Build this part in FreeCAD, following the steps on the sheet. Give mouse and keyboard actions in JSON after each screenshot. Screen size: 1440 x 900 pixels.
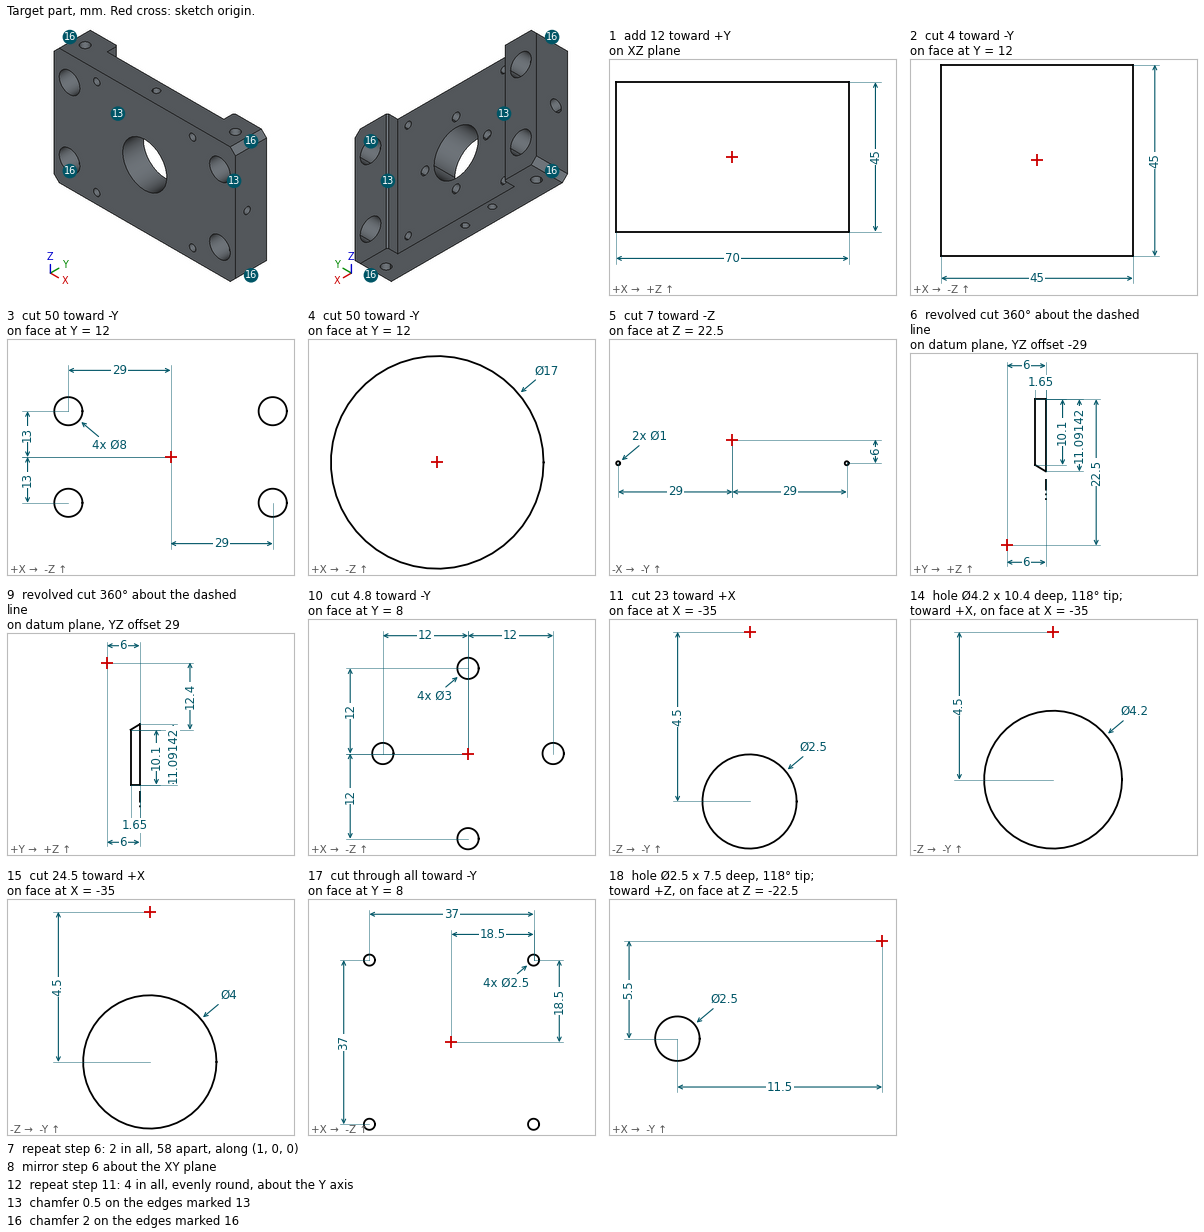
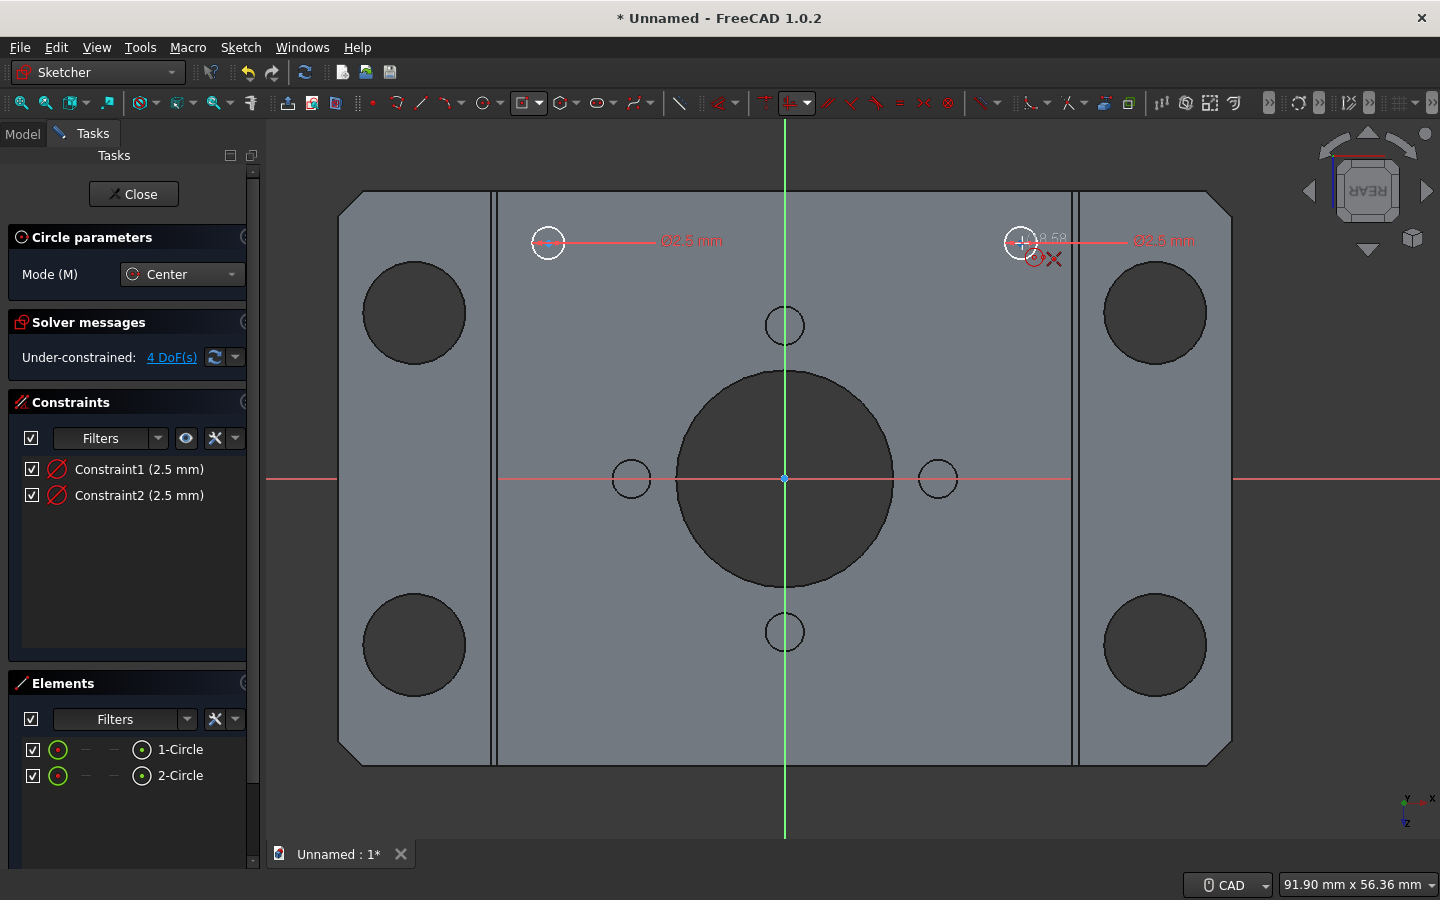
{"action": "scroll", "coordinate": [548, 715], "scroll_direction": "up", "scroll_amount": 2}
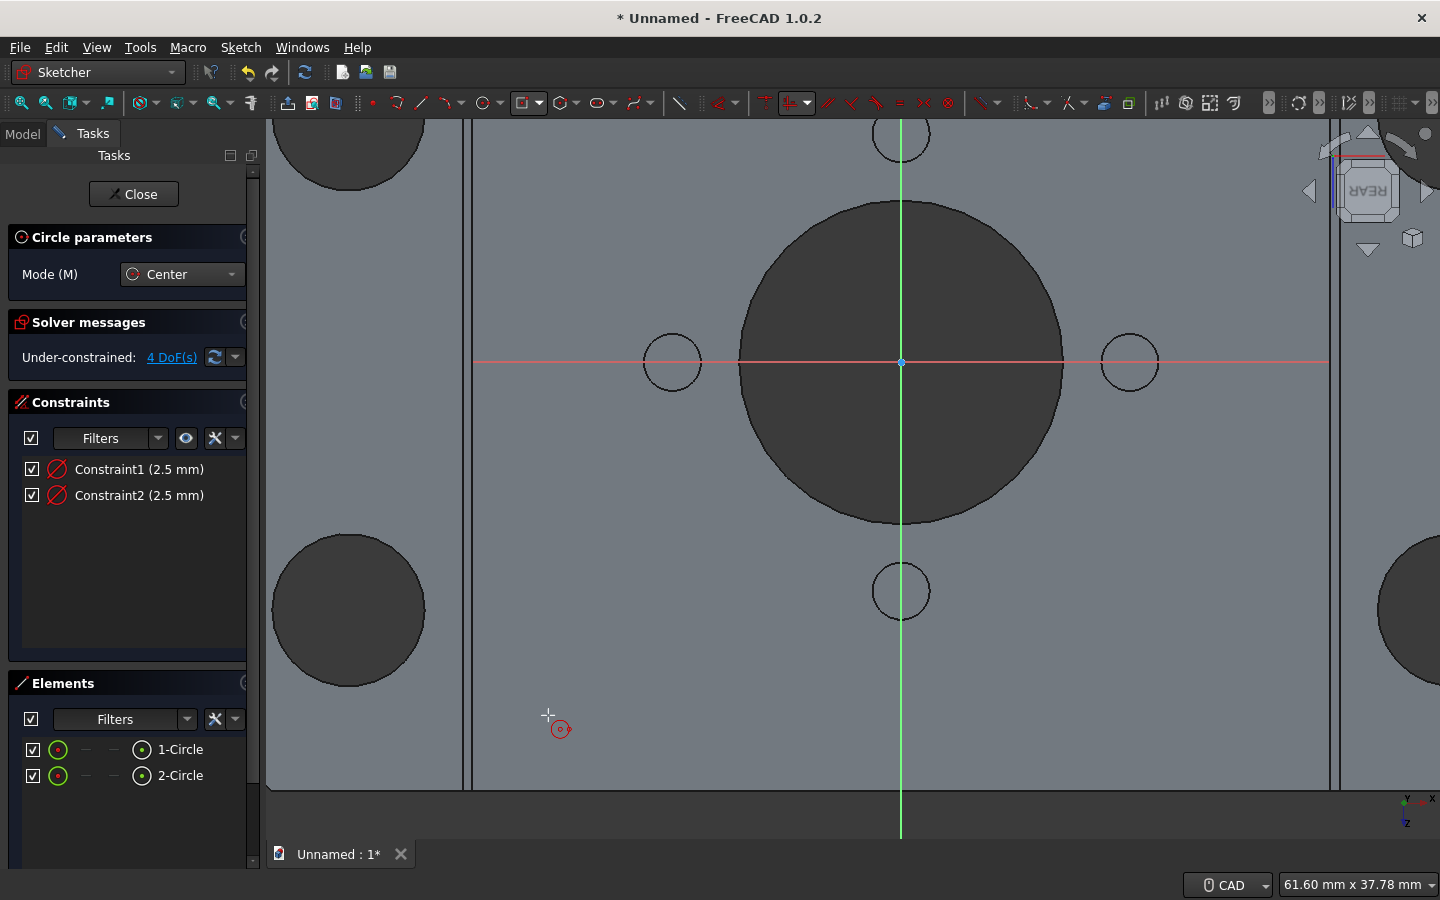
{"action": "left_click", "coordinate": [549, 715]}
{"action": "mouse_move", "coordinate": [565, 698]}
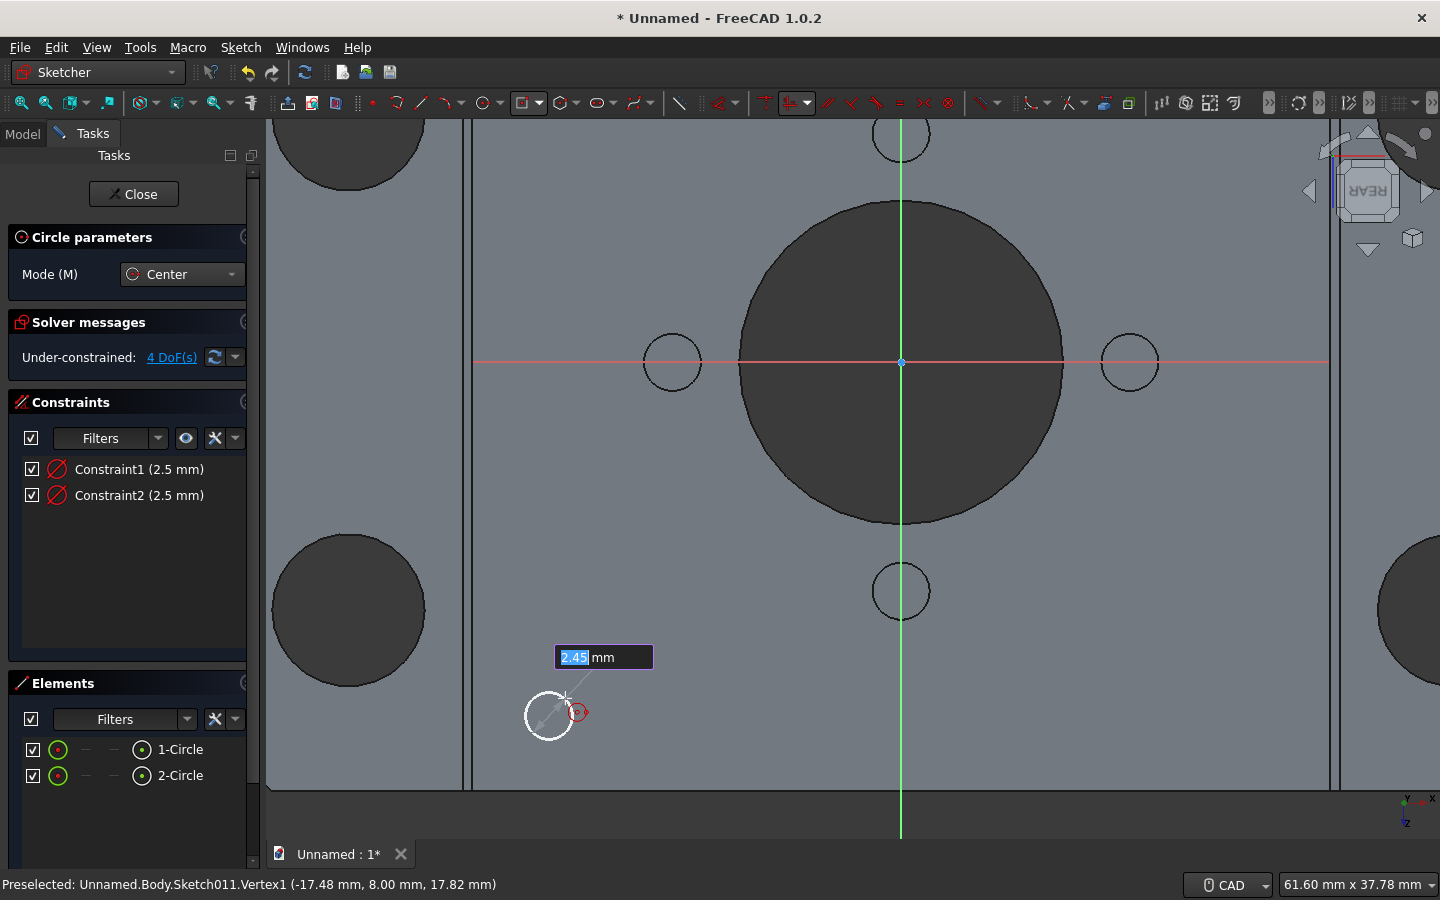
{"action": "type", "text": "2.5"}
{"action": "key", "text": "Return"}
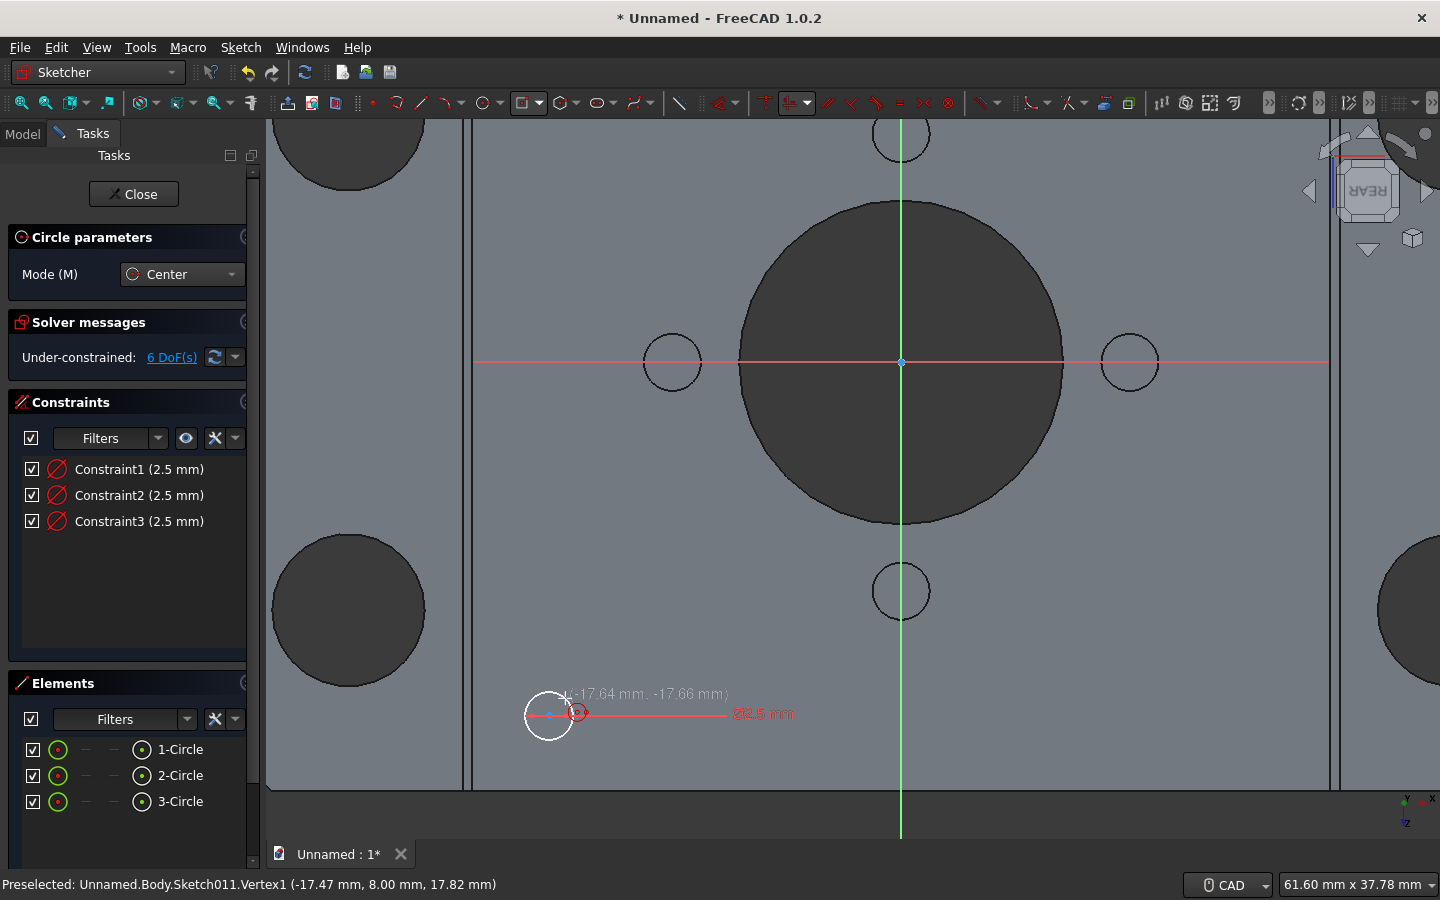
{"action": "left_click", "coordinate": [1254, 715]}
{"action": "mouse_move", "coordinate": [1271, 698]}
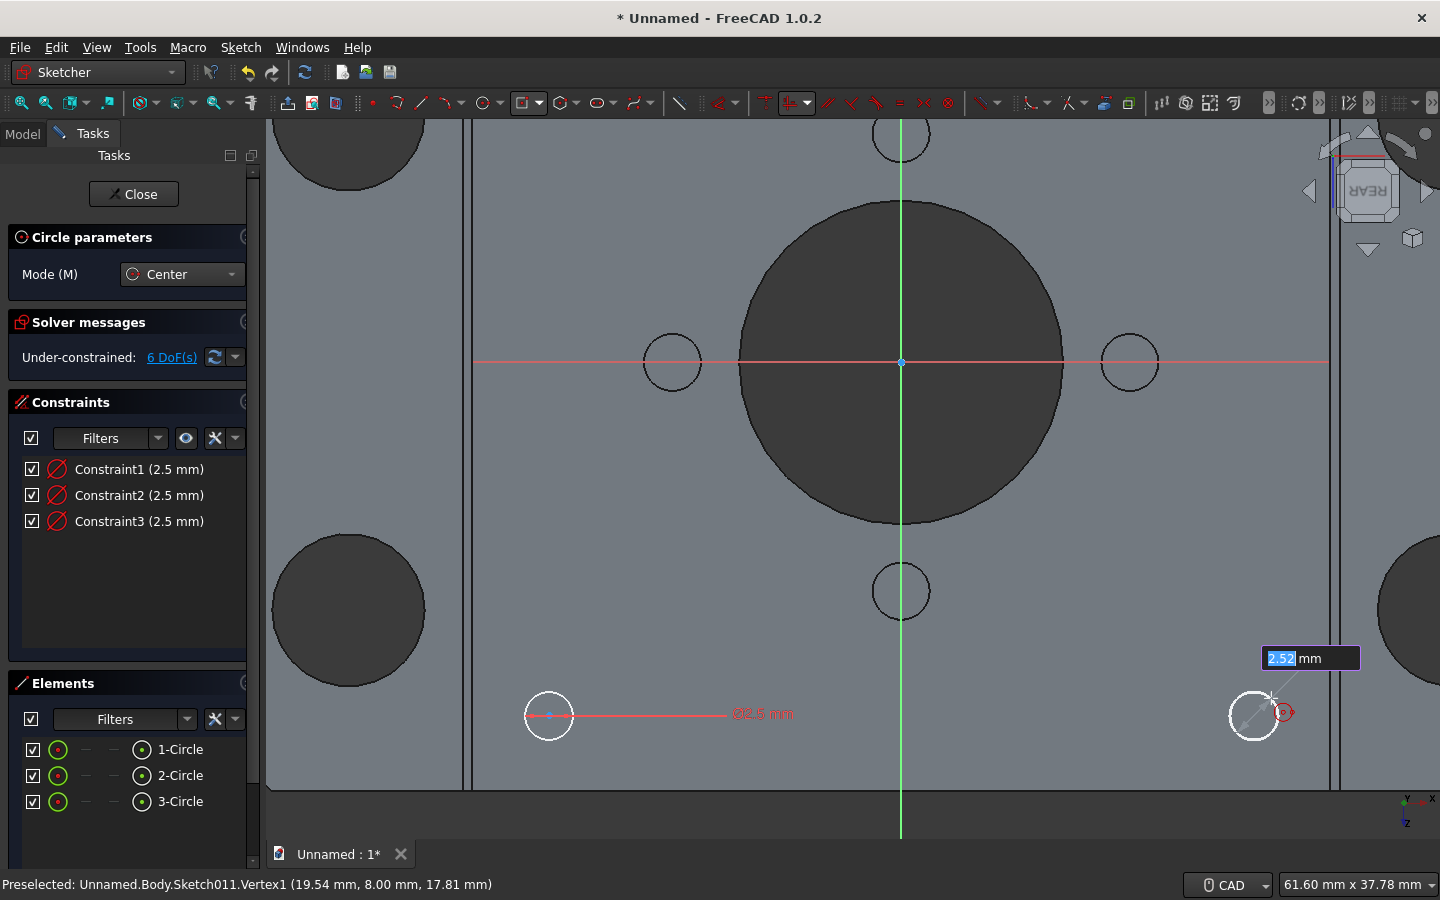
{"action": "type", "text": "2.5"}
{"action": "key", "text": "Return"}
{"action": "key", "text": "Escape"}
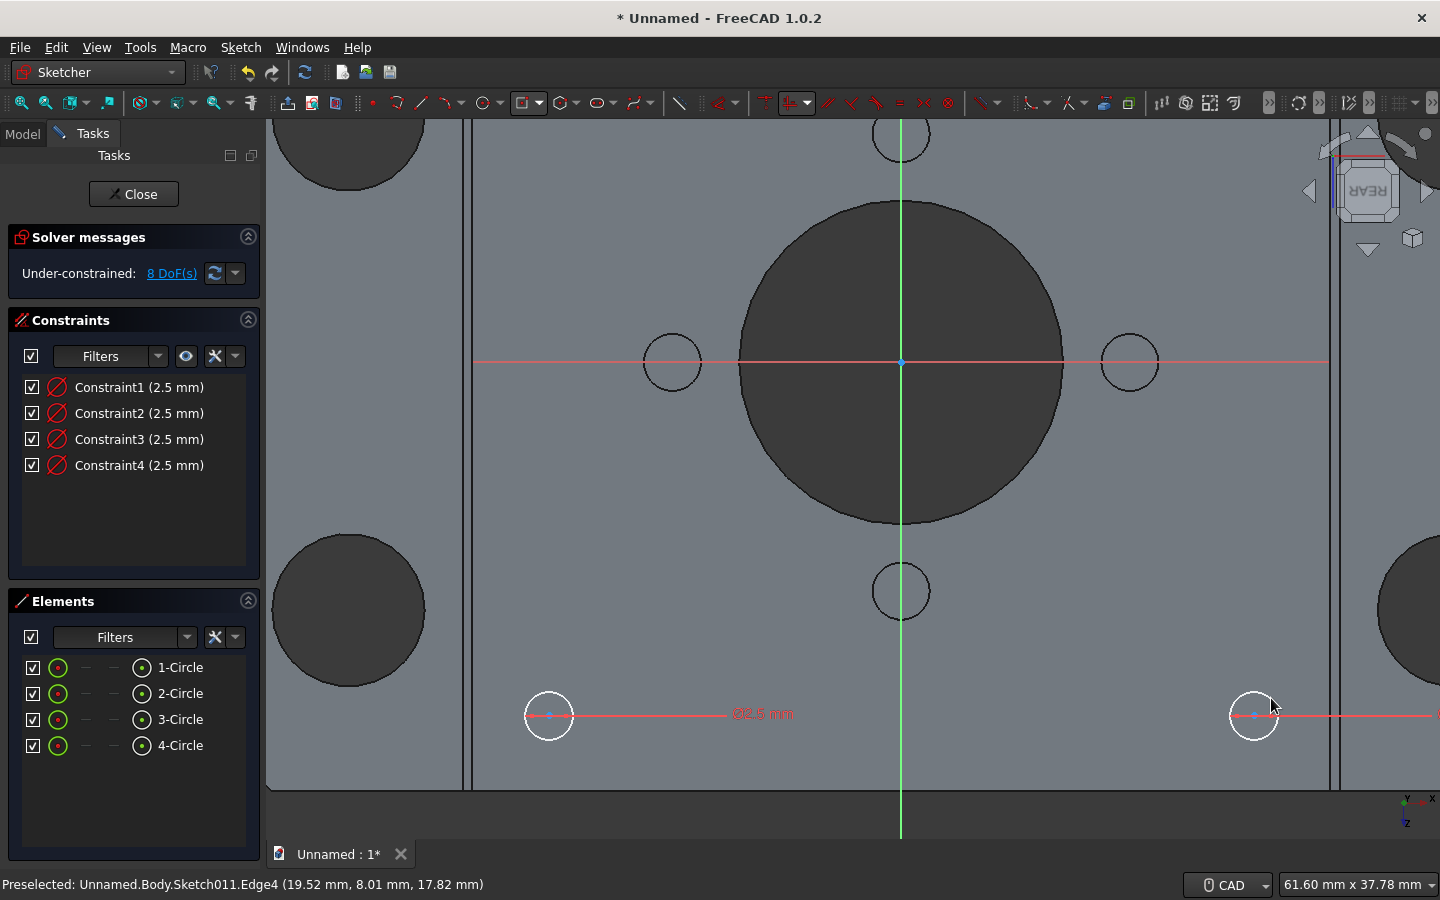
{"action": "scroll", "coordinate": [547, 716], "scroll_direction": "down", "scroll_amount": 2}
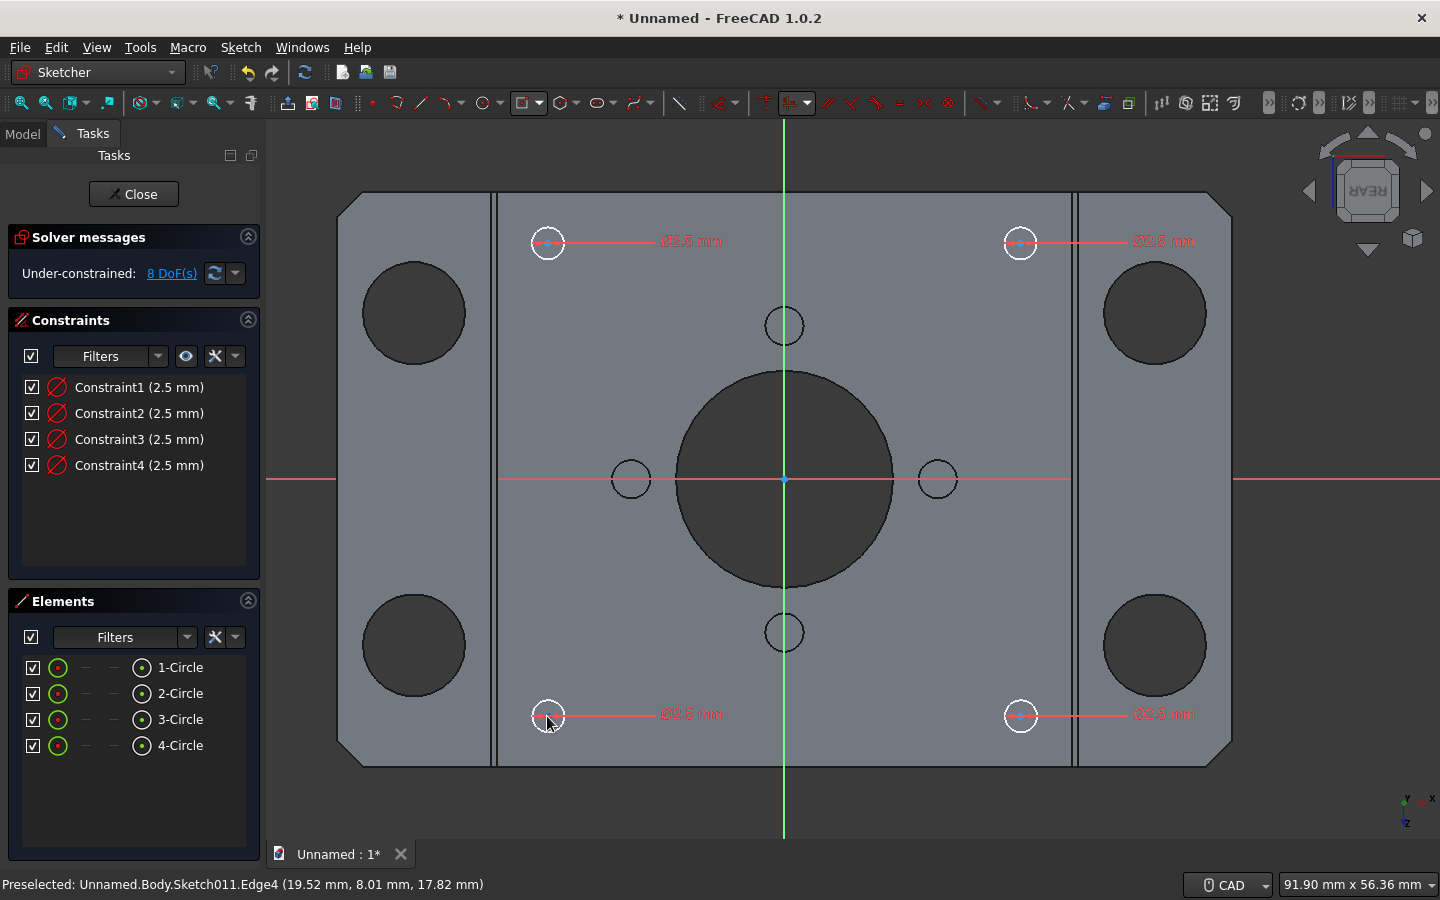
{"action": "left_click", "coordinate": [1021, 243]}